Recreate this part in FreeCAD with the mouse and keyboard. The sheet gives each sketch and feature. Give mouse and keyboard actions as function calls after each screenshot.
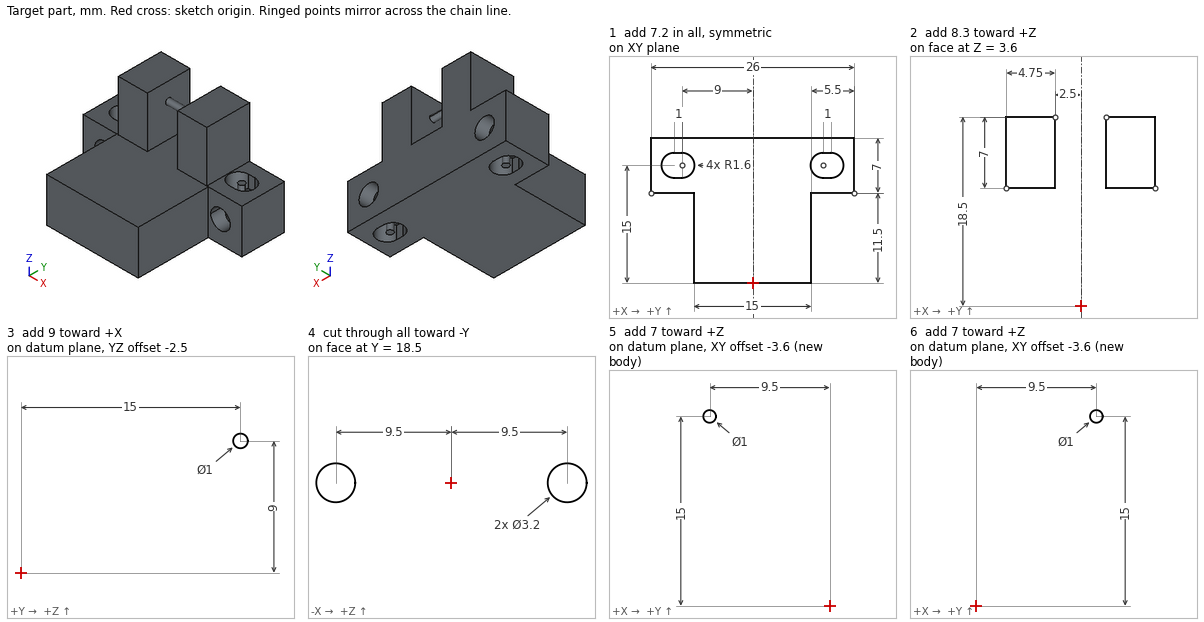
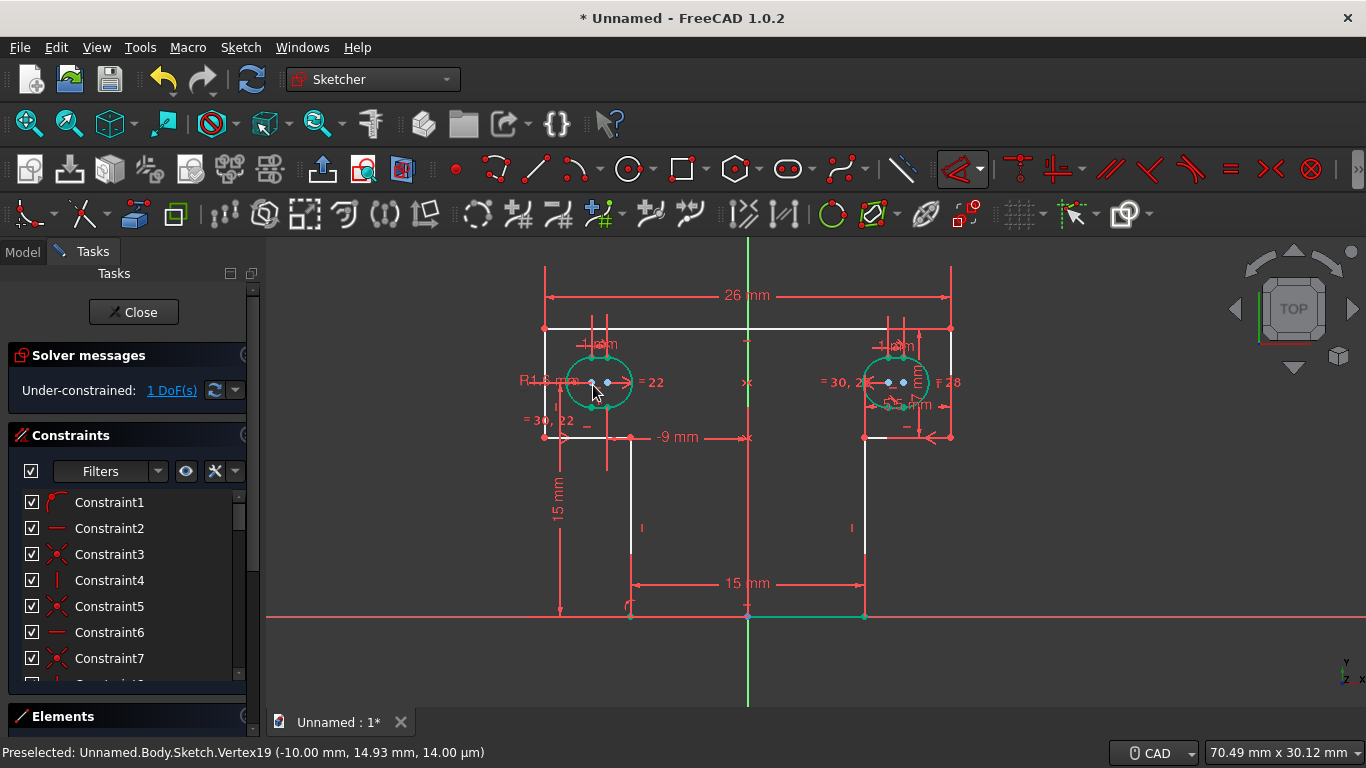
click(865, 563)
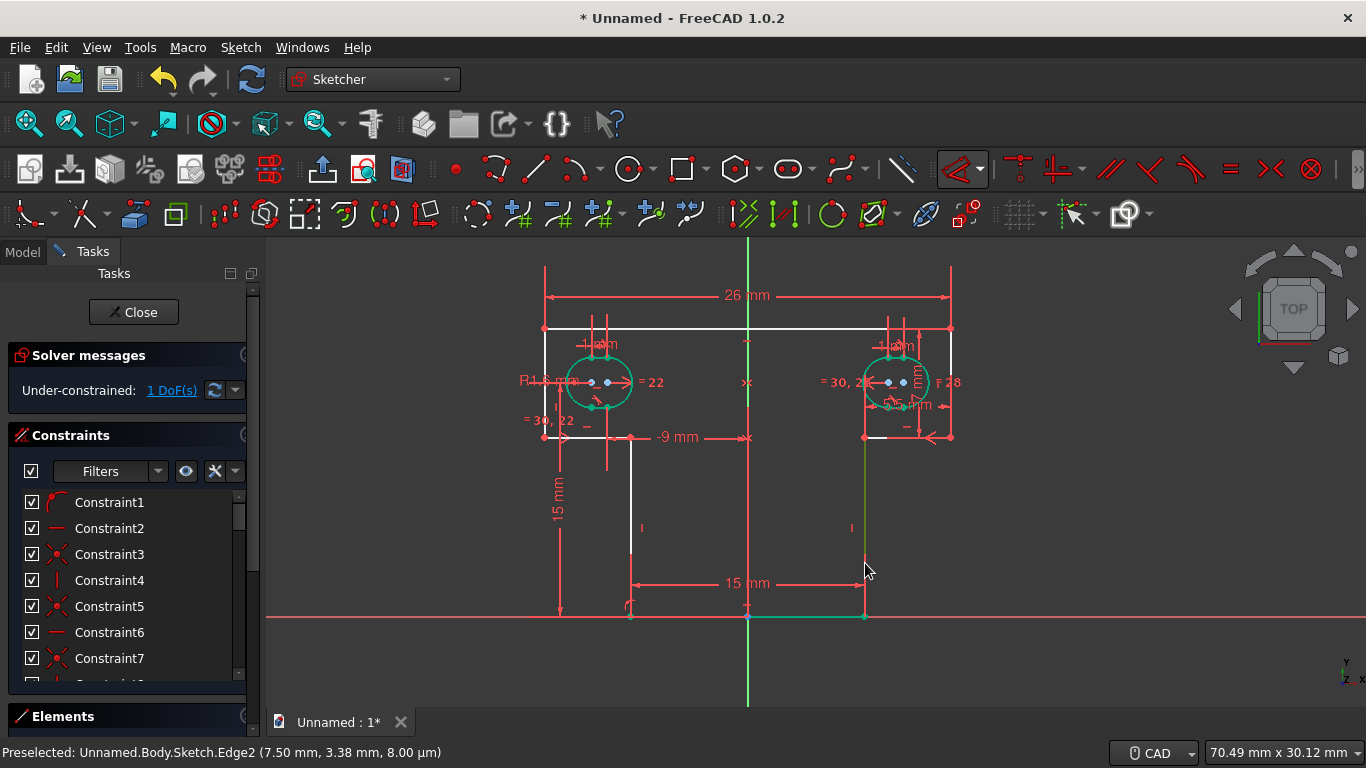
key(i)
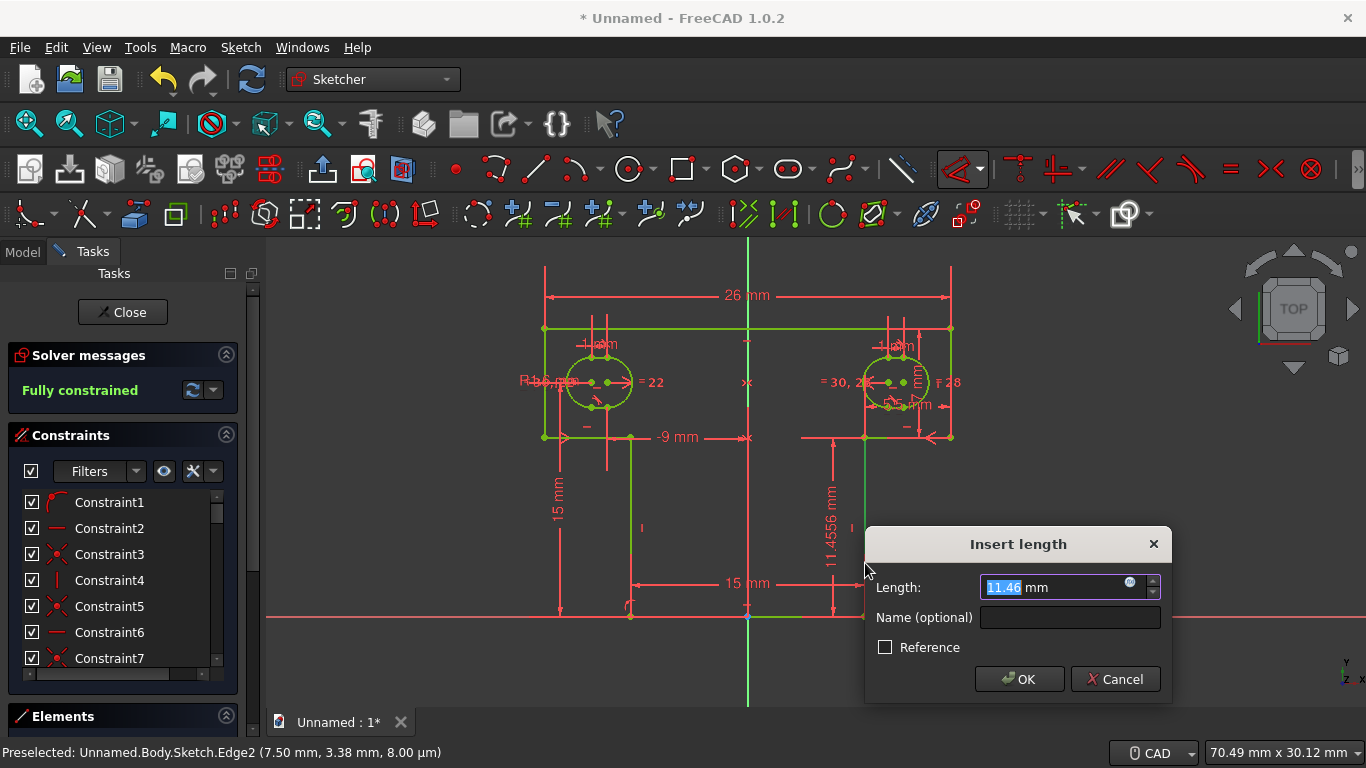
text(11.5)
key(Return)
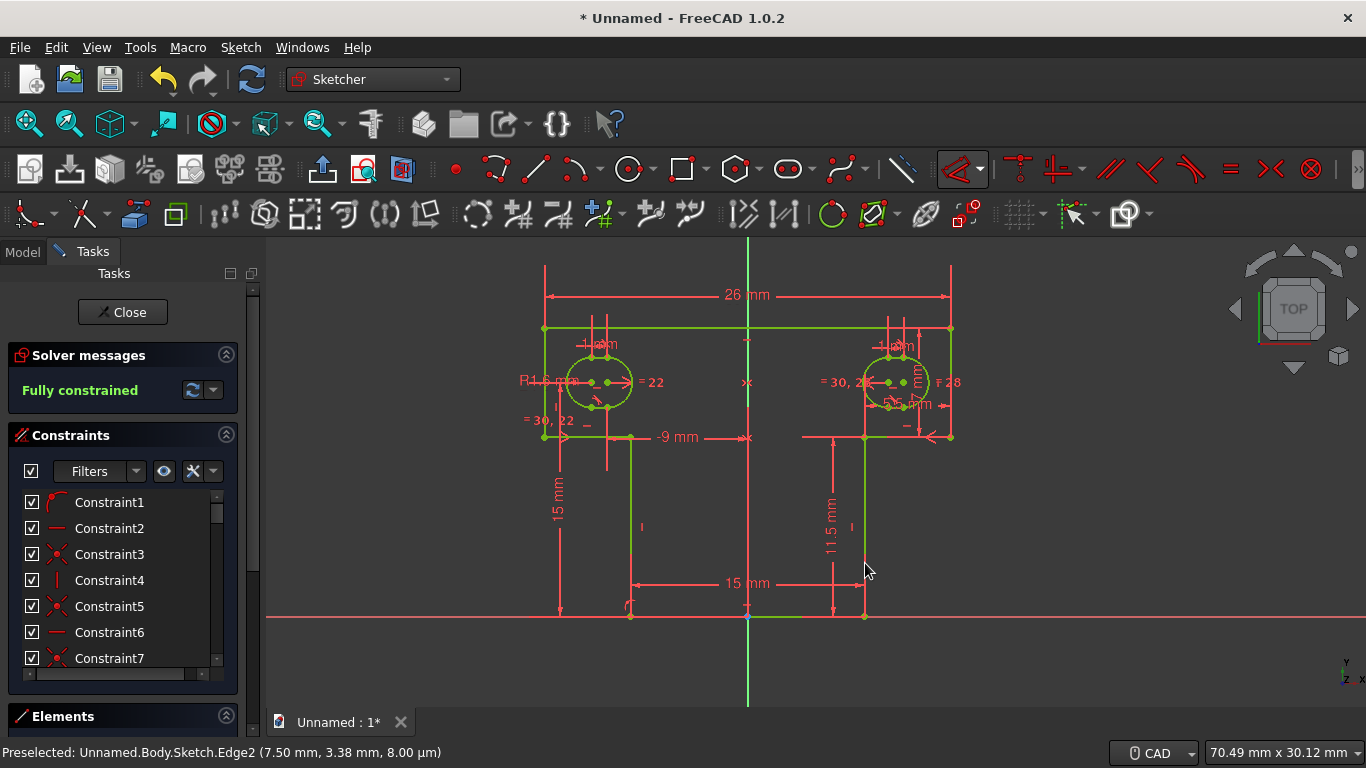
click(123, 312)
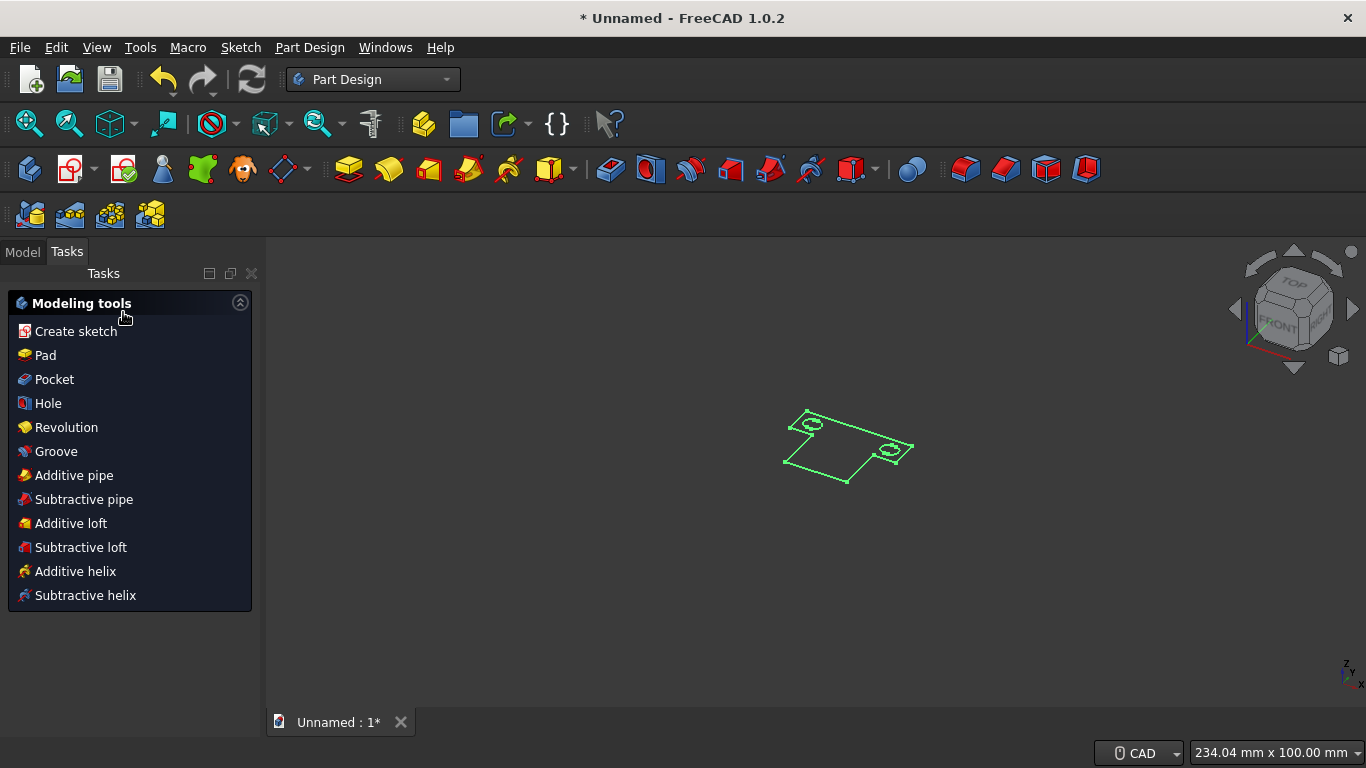
click(350, 170)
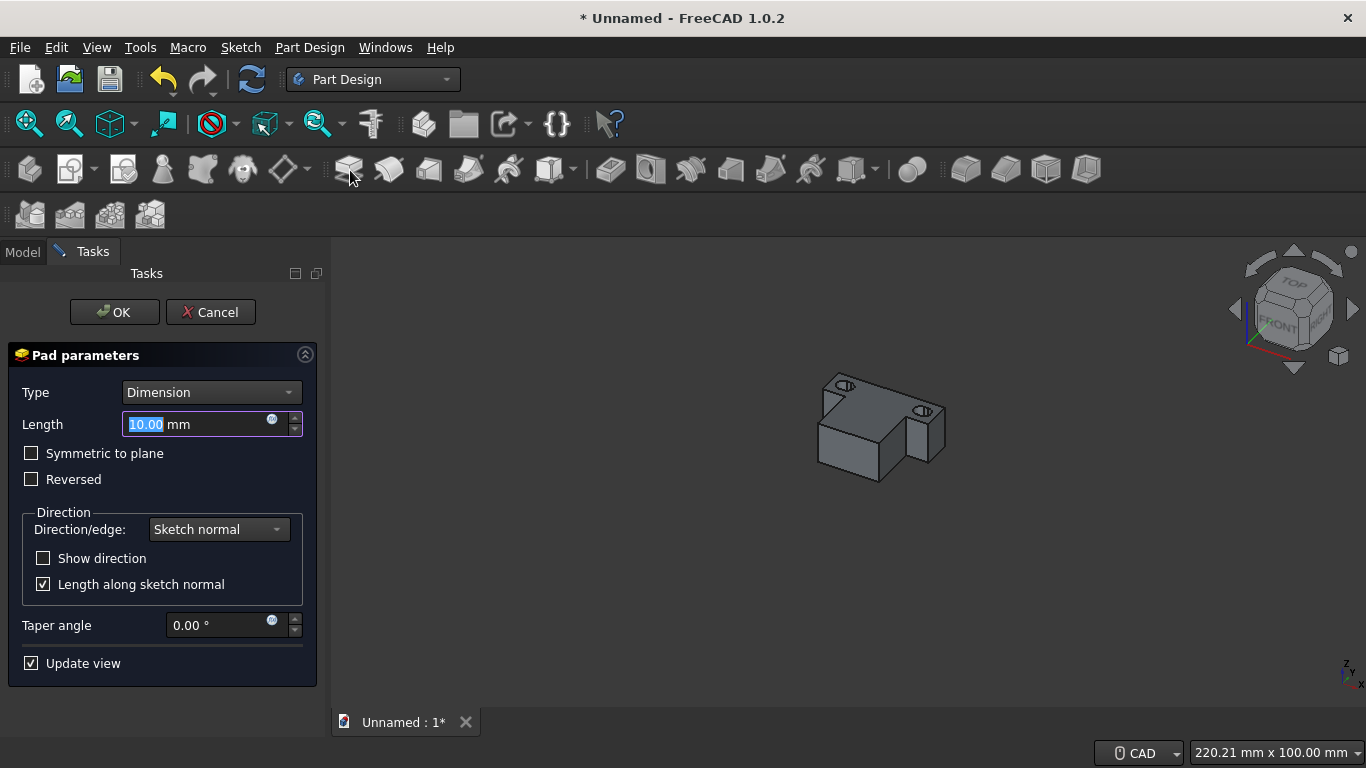
text(7.2)
key(Tab)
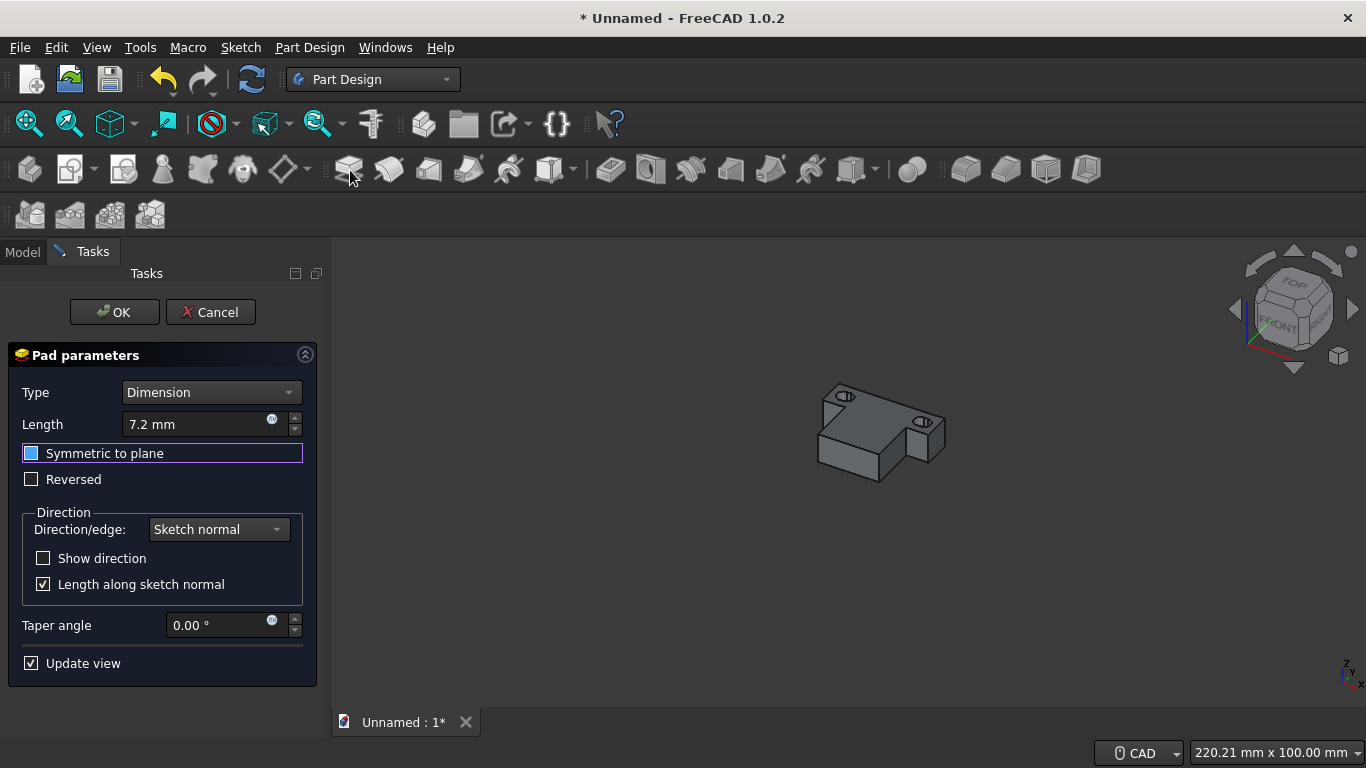
click(30, 453)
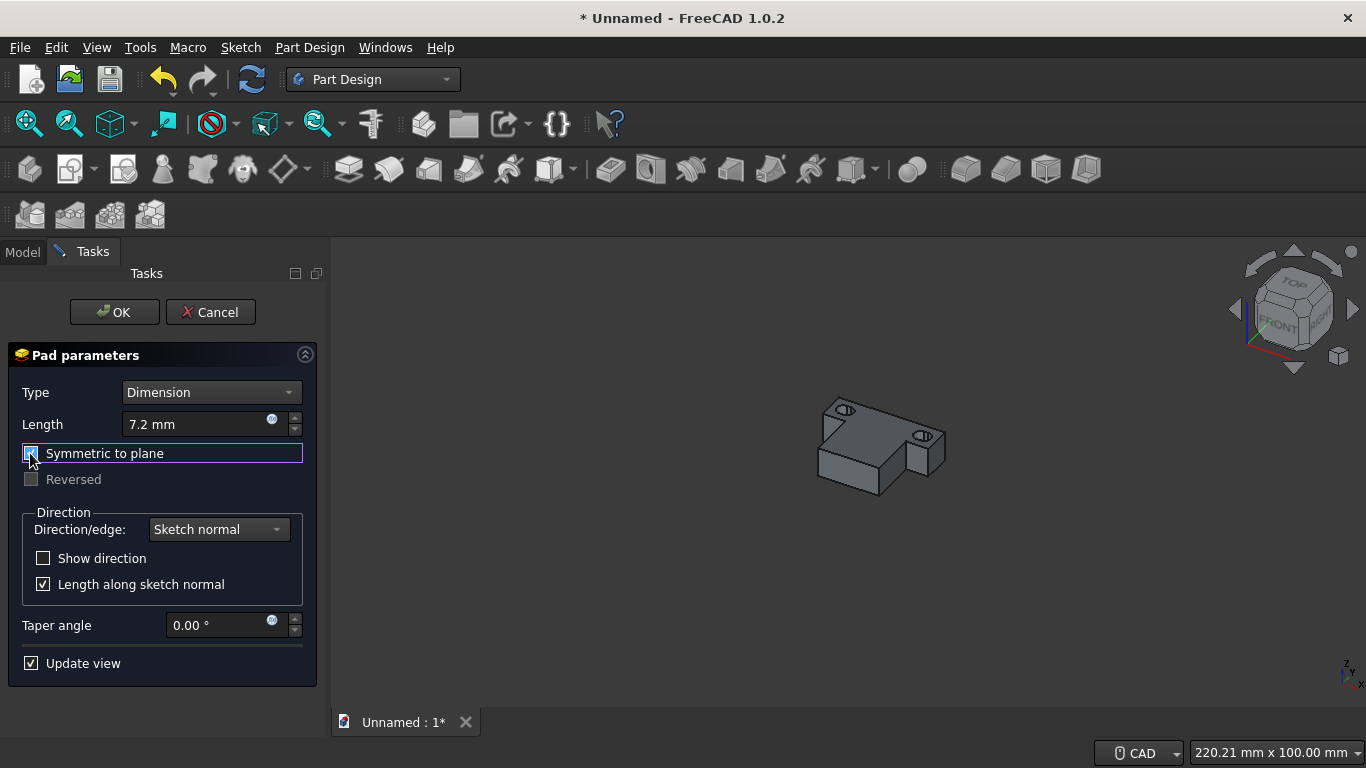
click(115, 312)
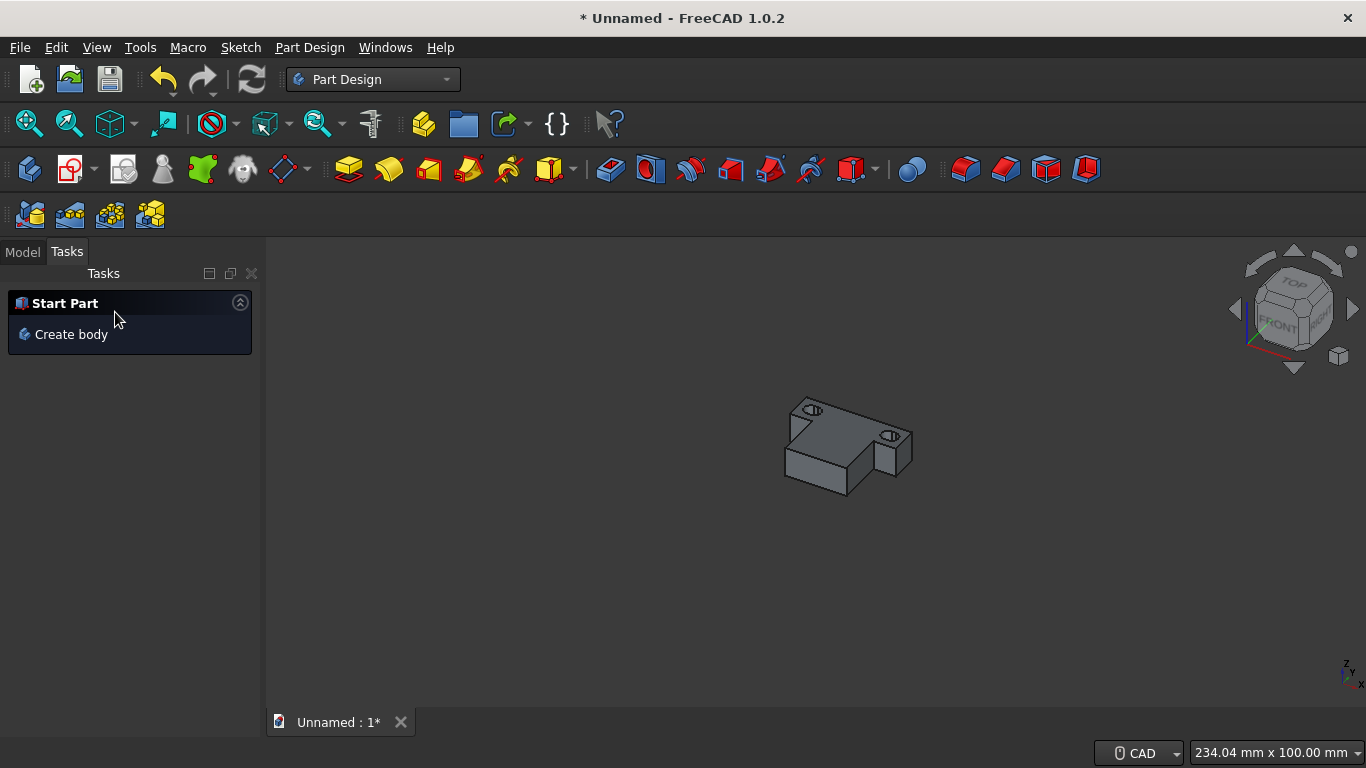
key(v)
key(f)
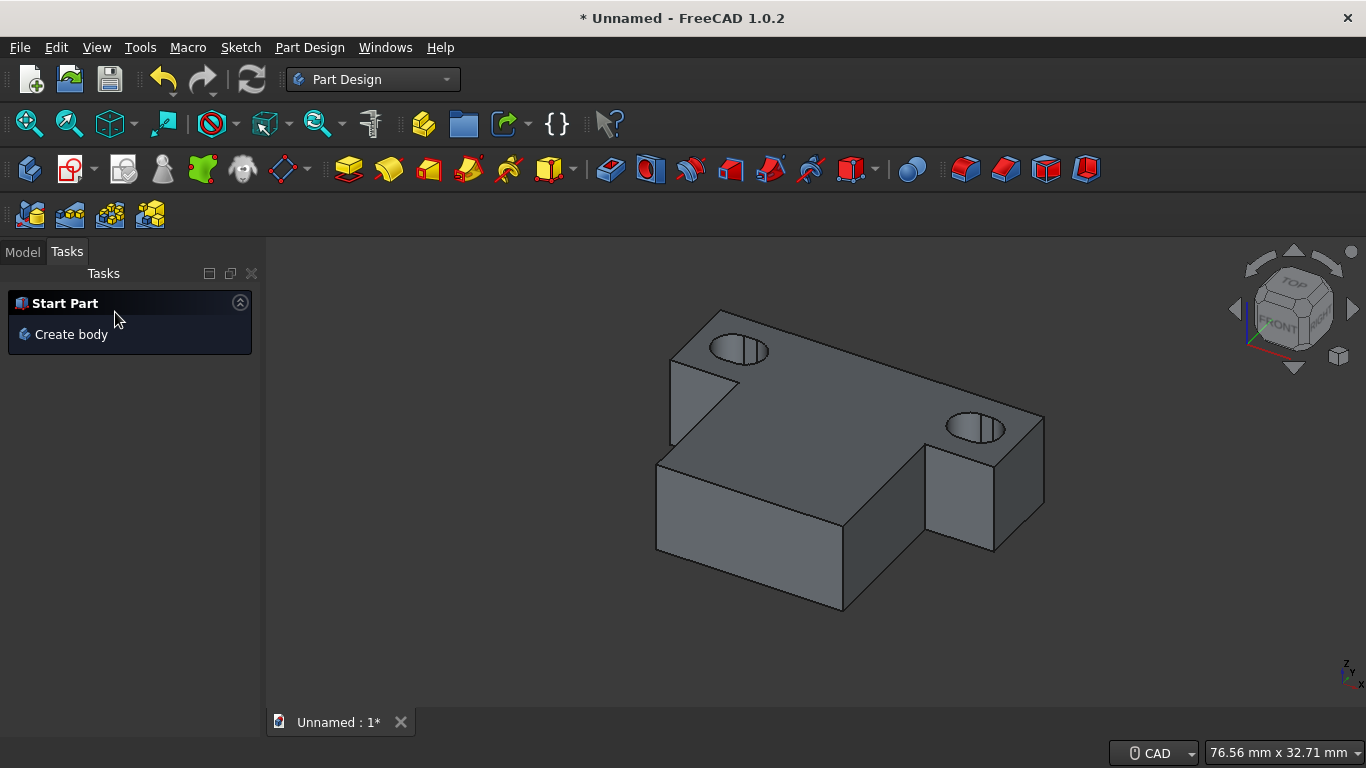
click(816, 429)